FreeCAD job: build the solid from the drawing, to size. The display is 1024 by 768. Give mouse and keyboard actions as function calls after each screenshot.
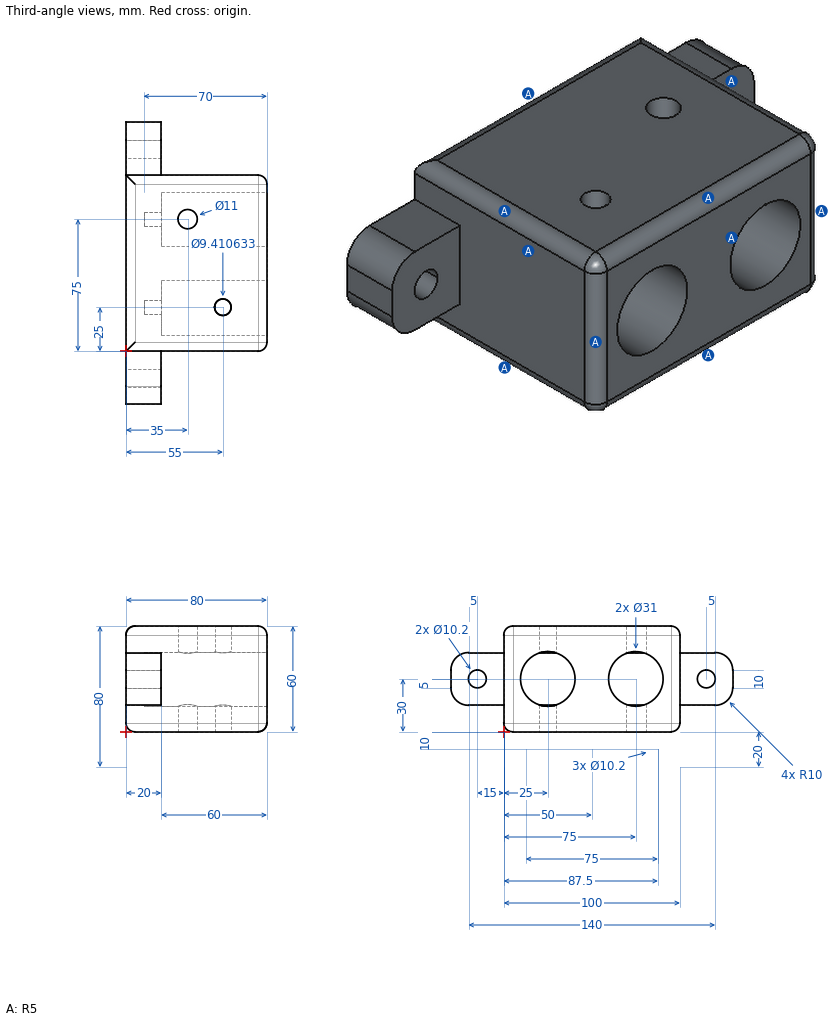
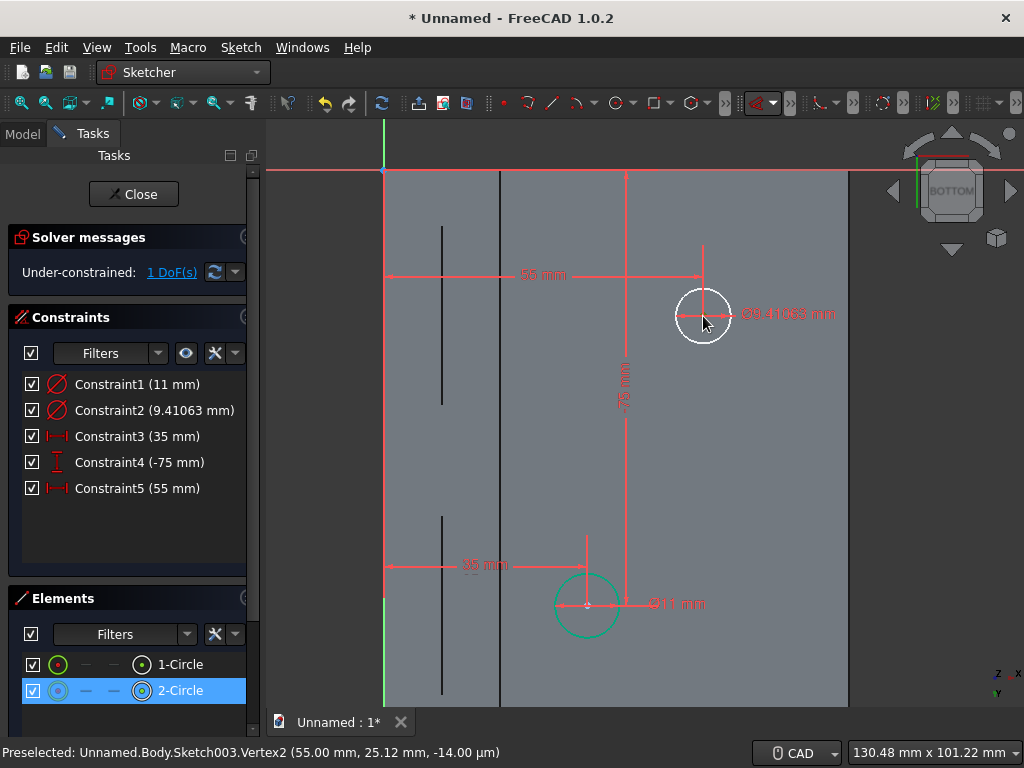
key(i)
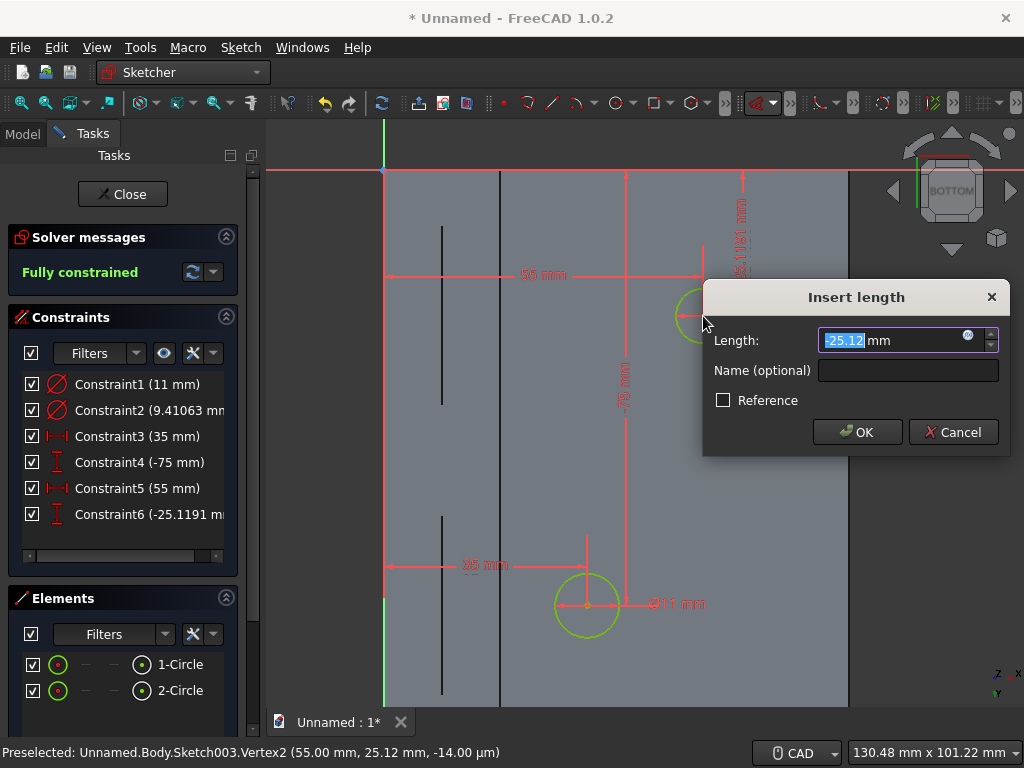
text(-25)
key(Return)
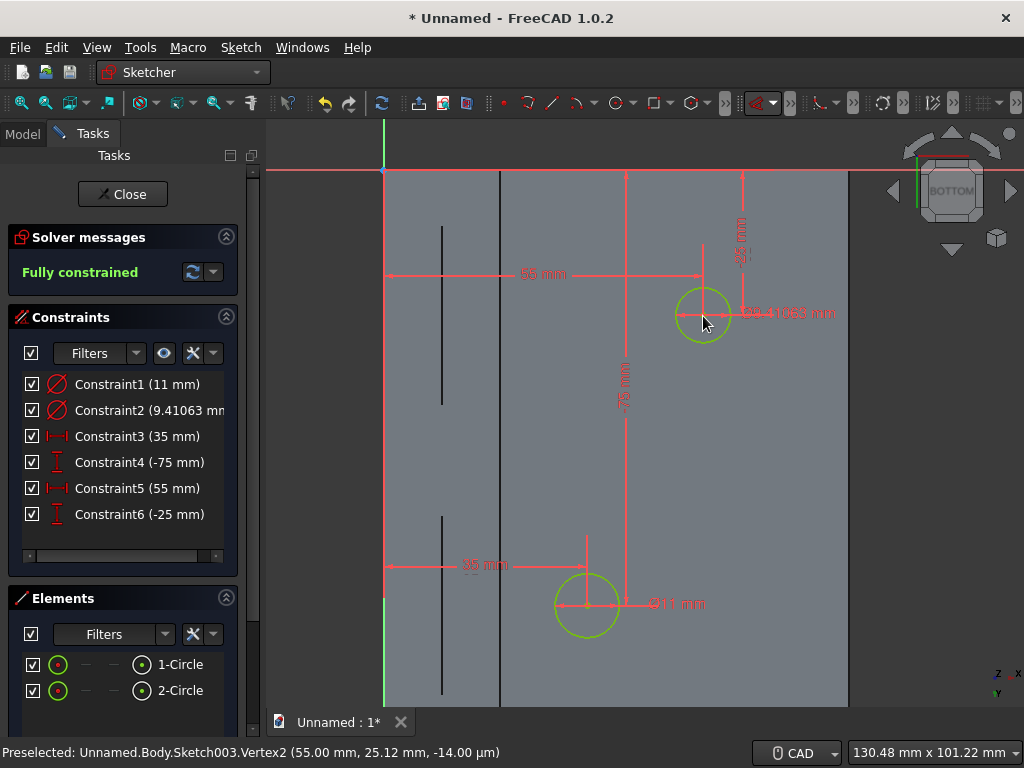
click(123, 194)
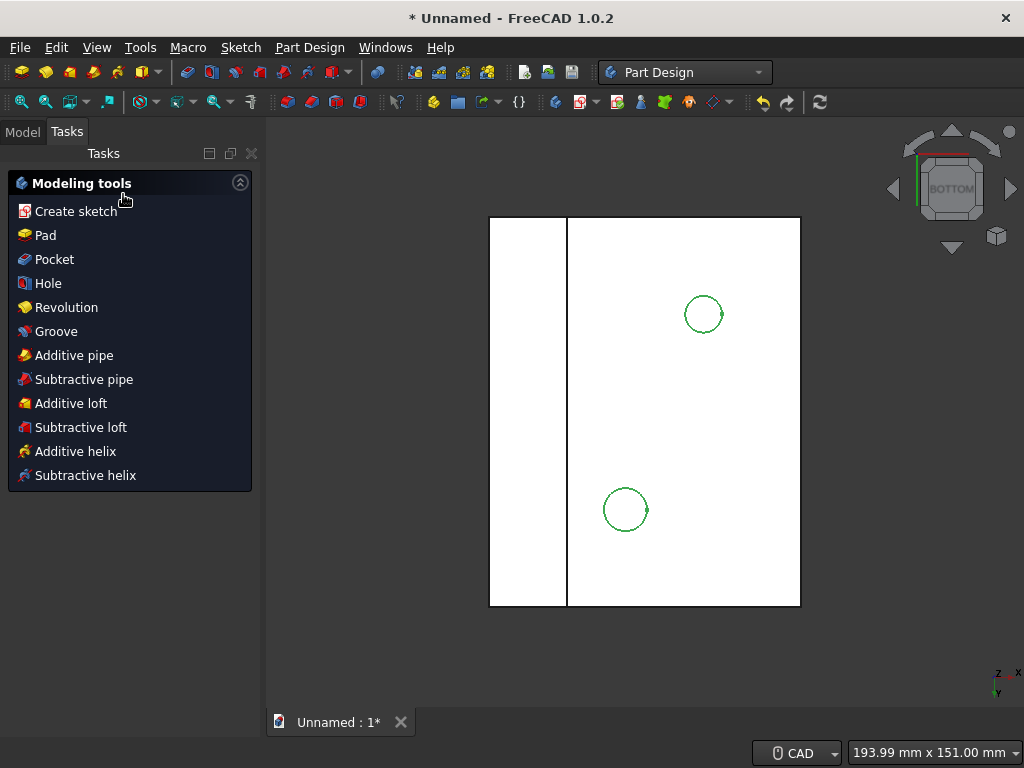
click(188, 72)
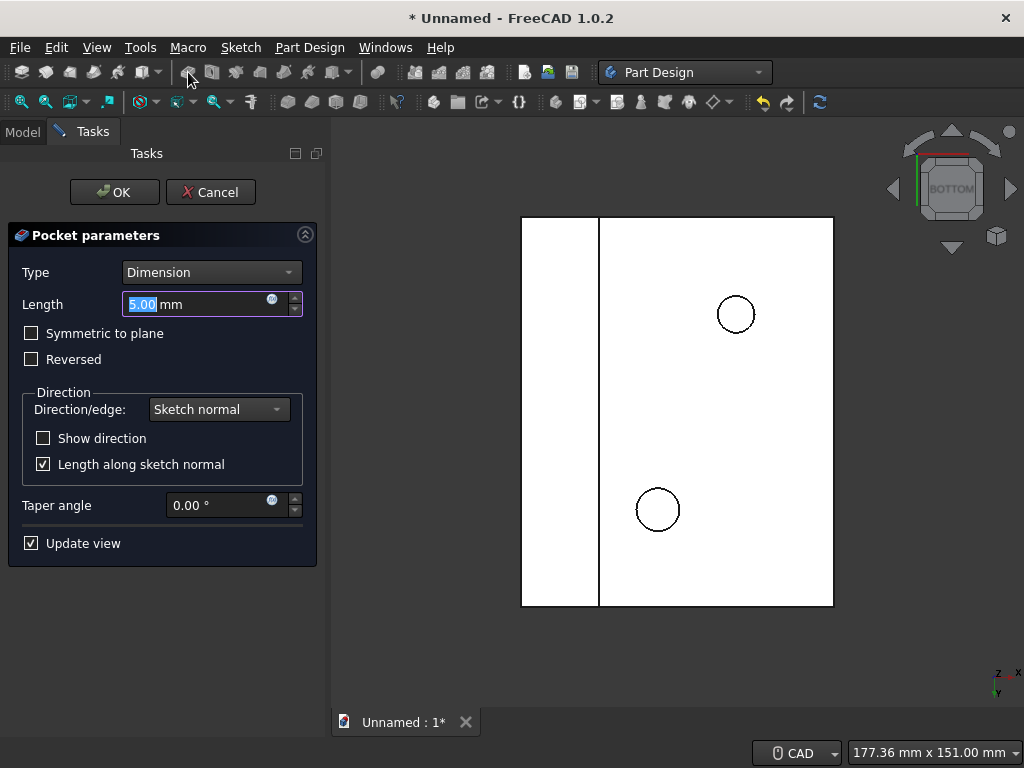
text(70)
key(Tab)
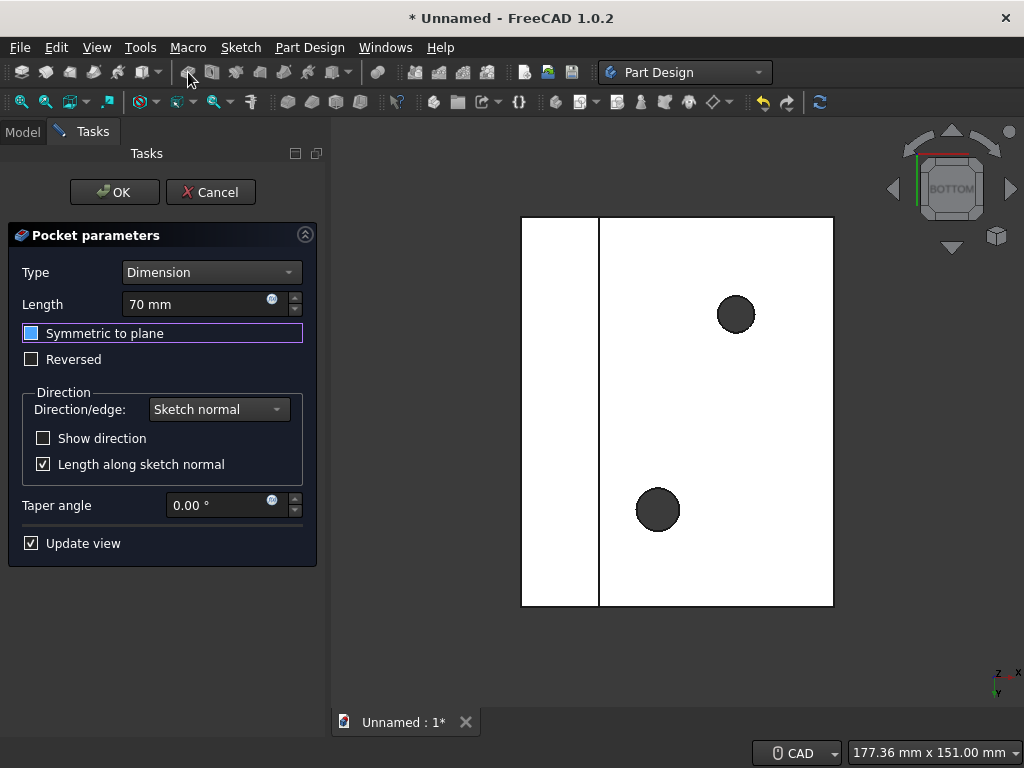
click(115, 192)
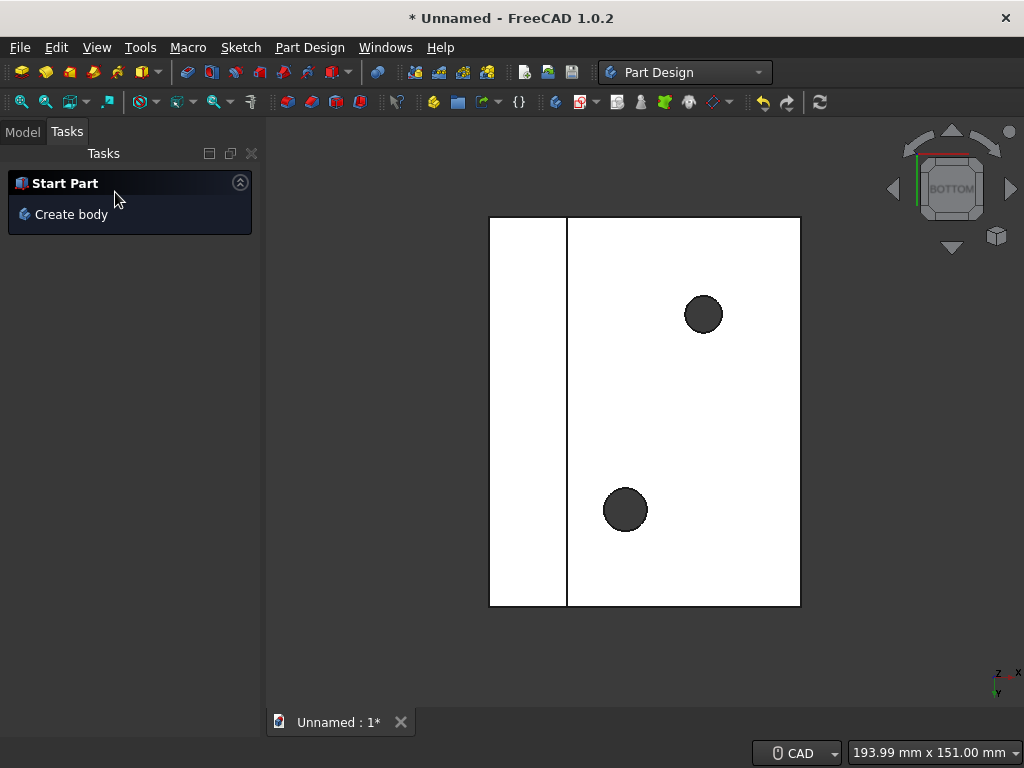
click(580, 102)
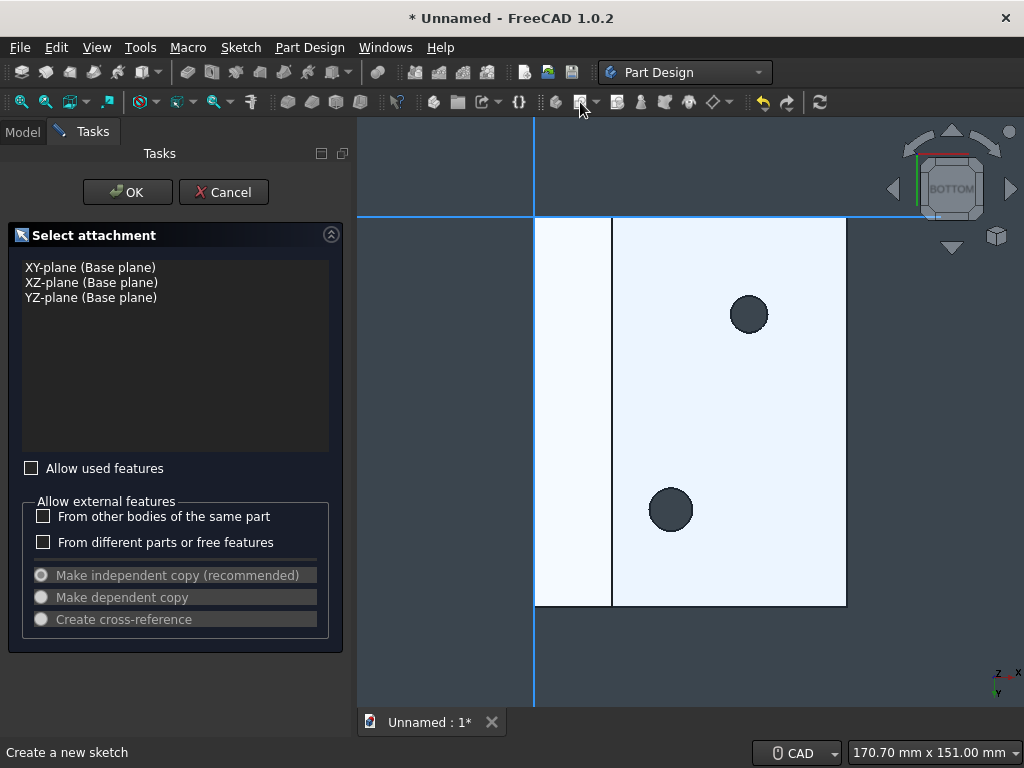
click(82, 298)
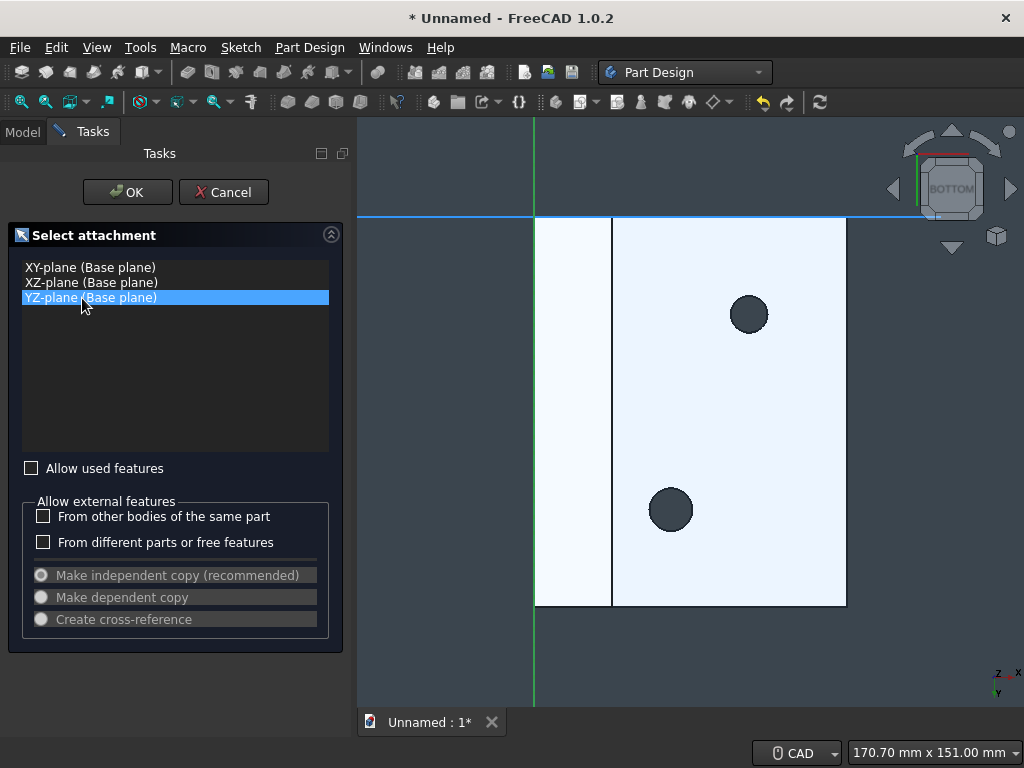
click(128, 192)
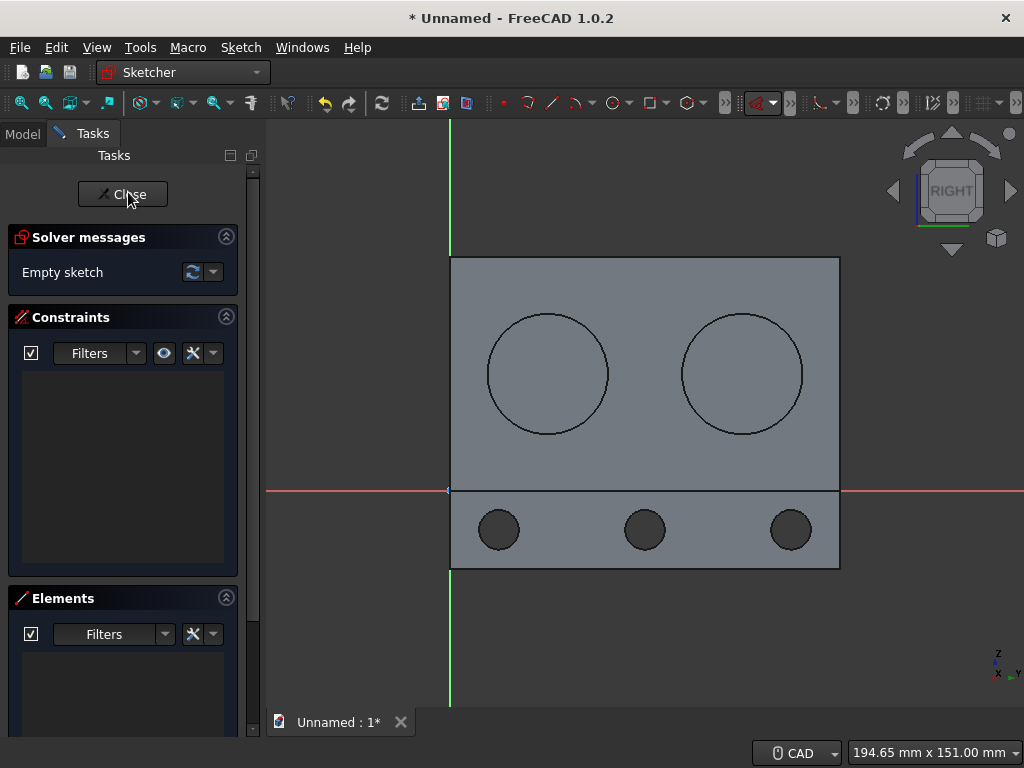
key(q)
key(s)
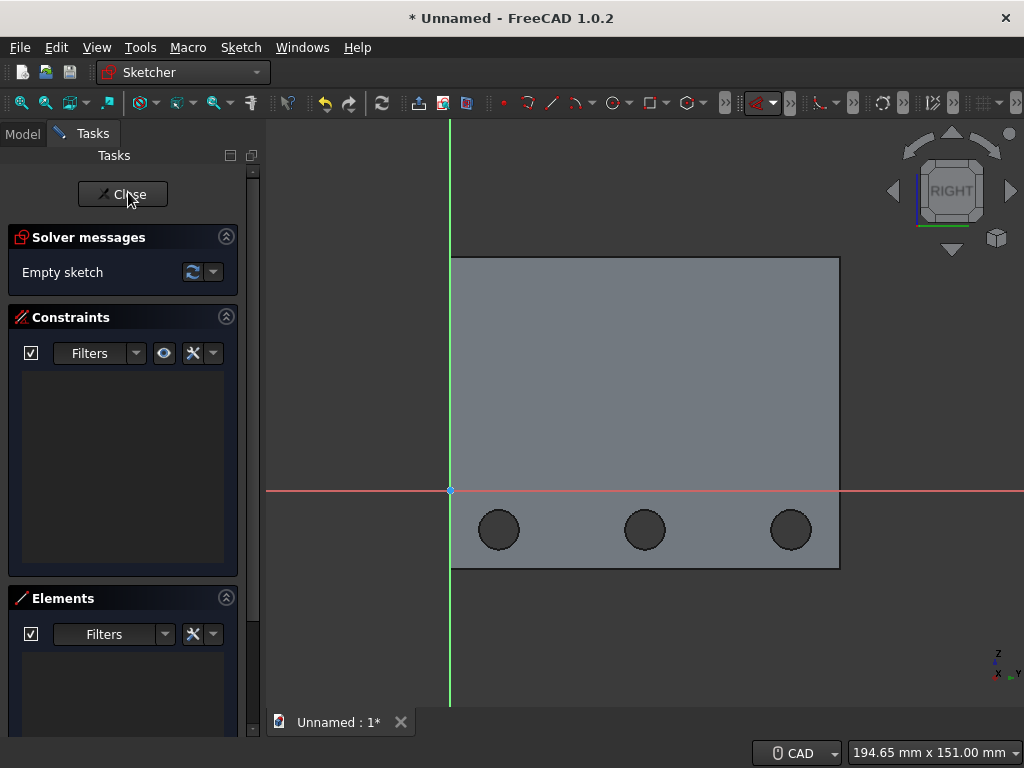
scroll(437, 433, down, 2)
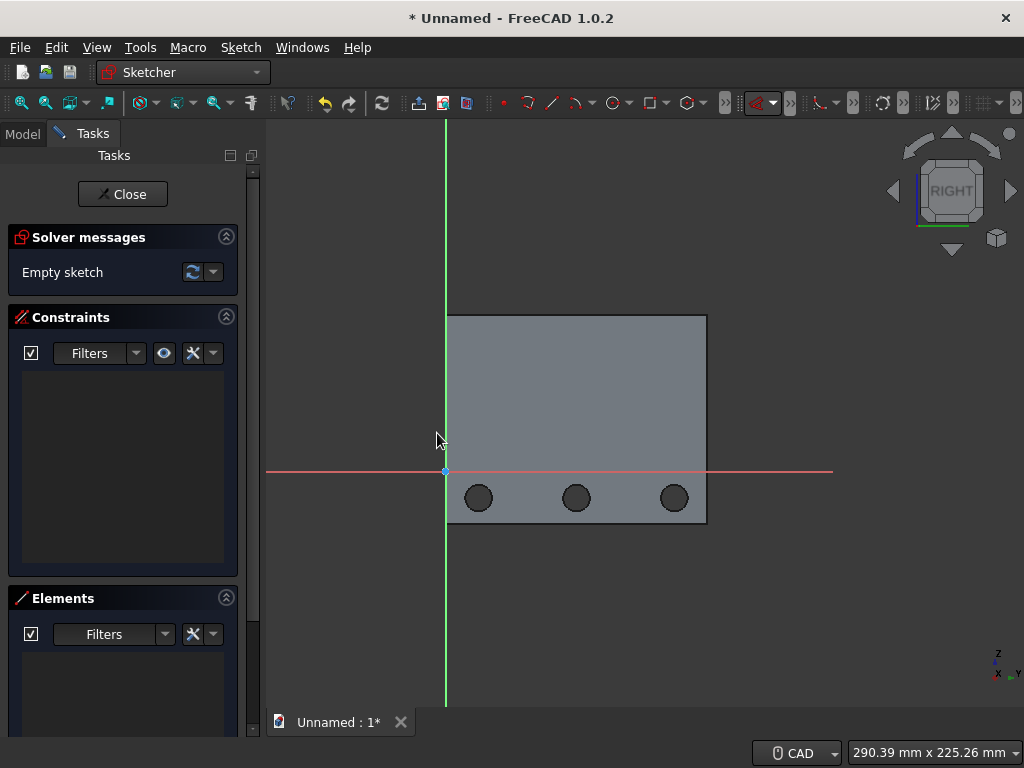
key(g)
key(l)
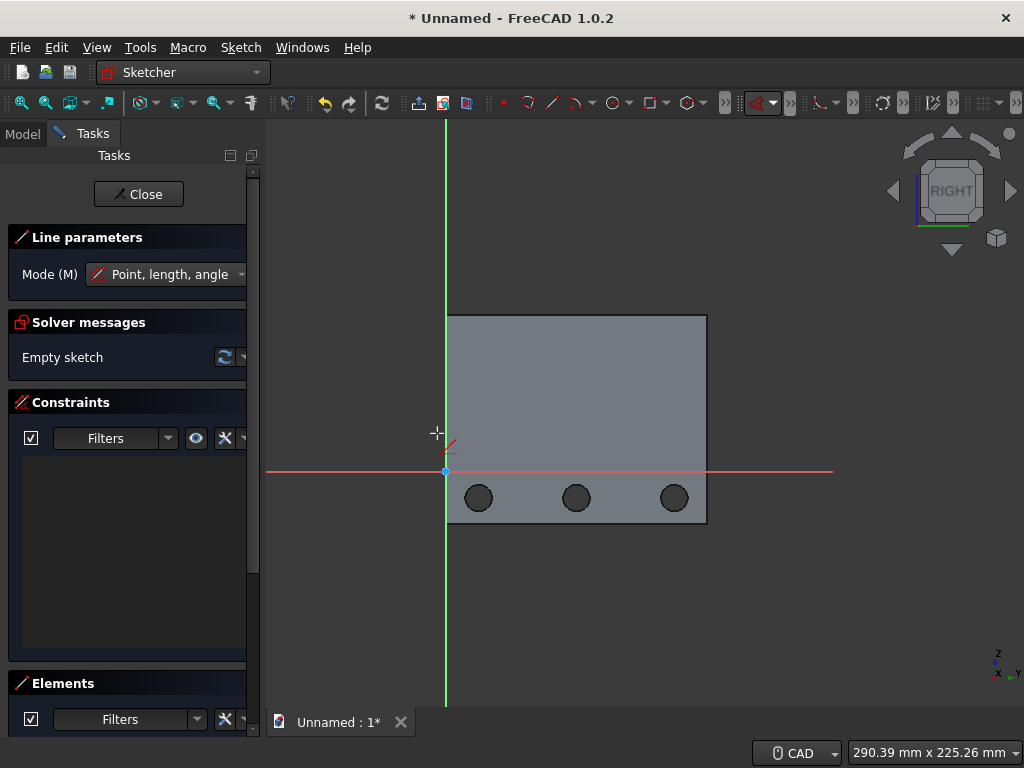
click(785, 381)
click(785, 407)